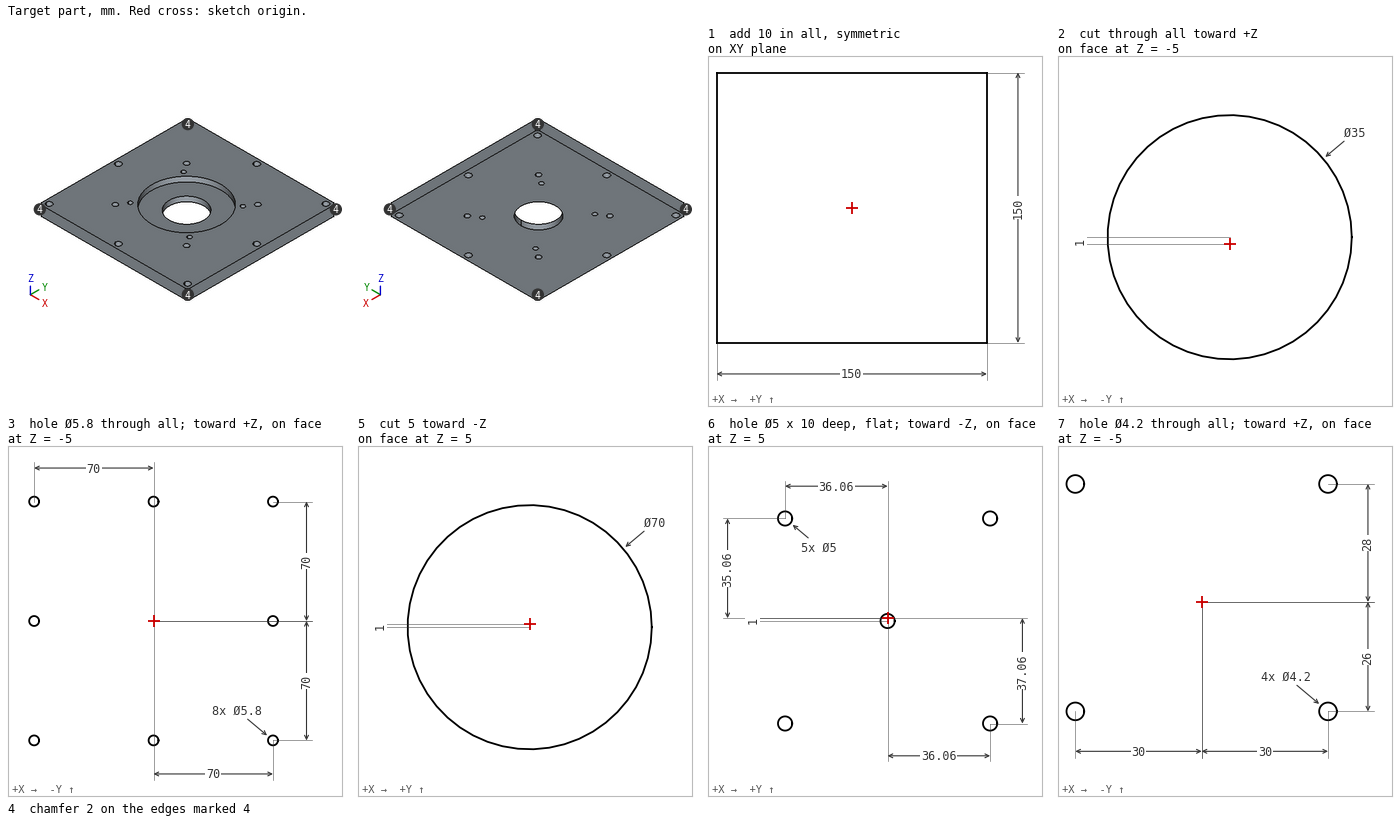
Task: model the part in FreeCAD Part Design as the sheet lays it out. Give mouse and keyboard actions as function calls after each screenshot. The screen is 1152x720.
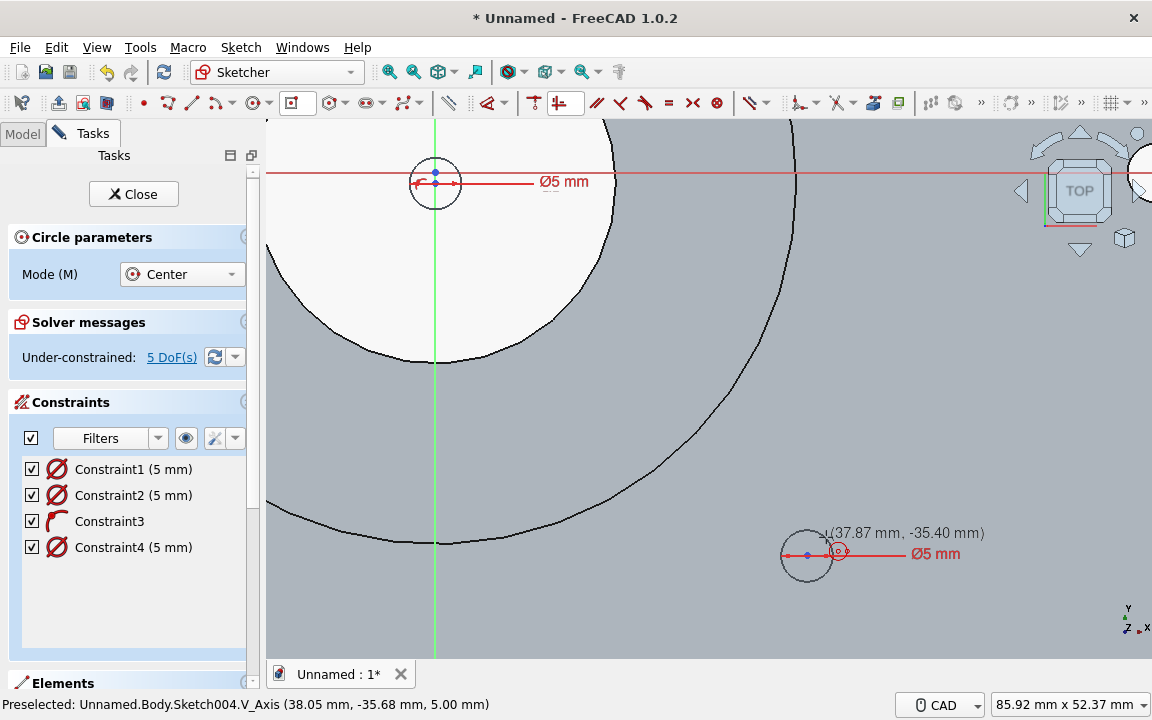
scroll(808, 557, down, 4)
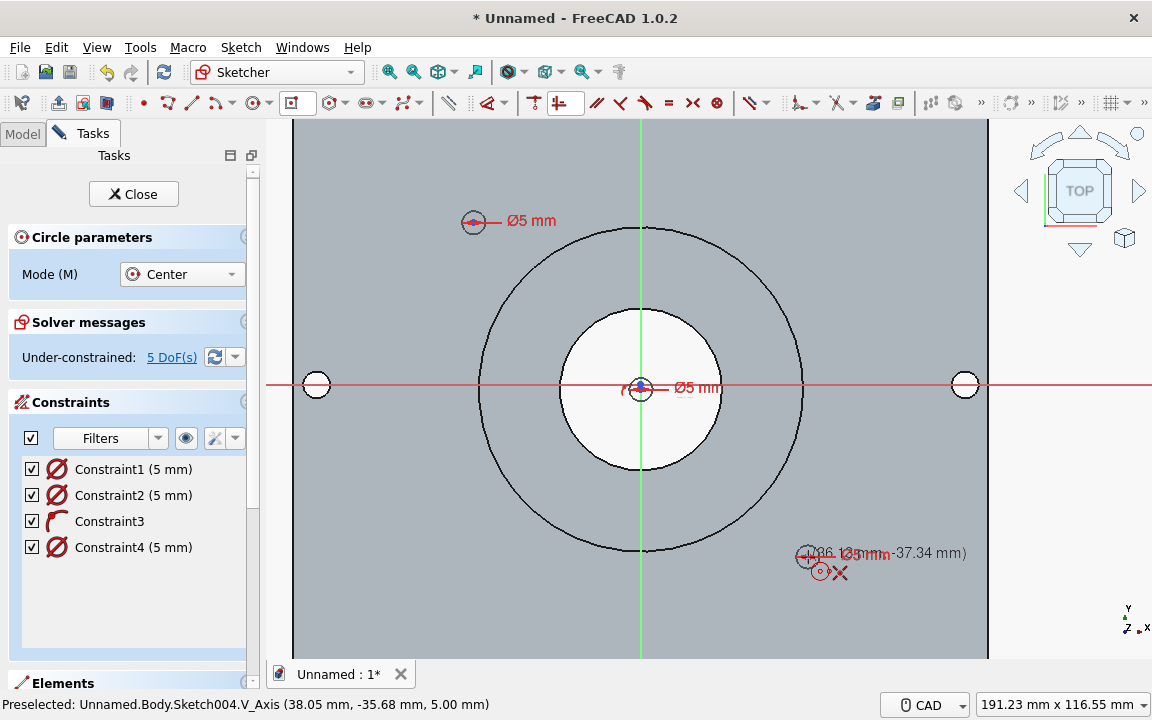
scroll(808, 222, up, 4)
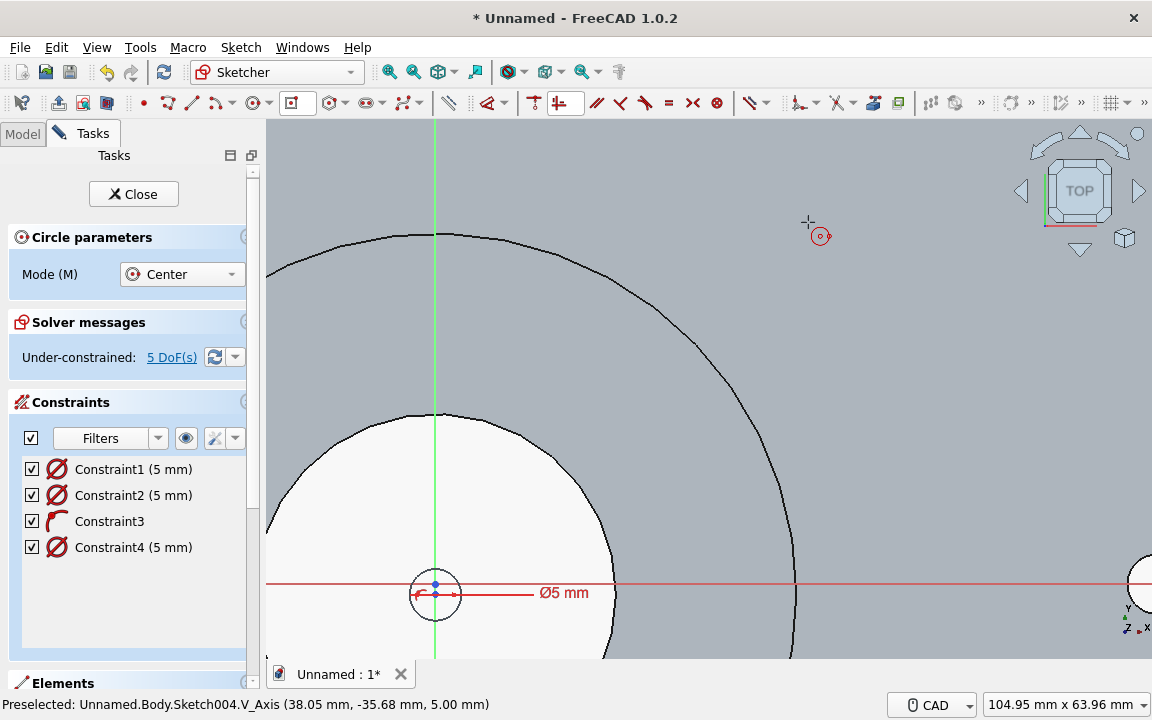
click(807, 223)
move(826, 205)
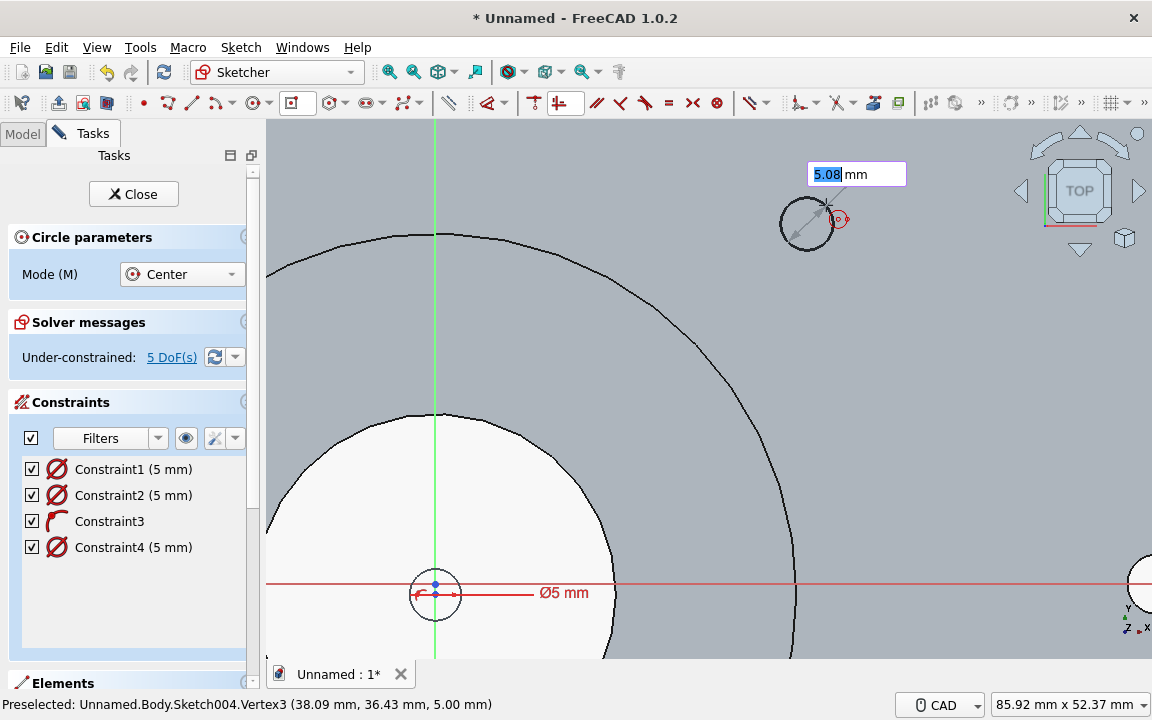
text(5)
key(Return)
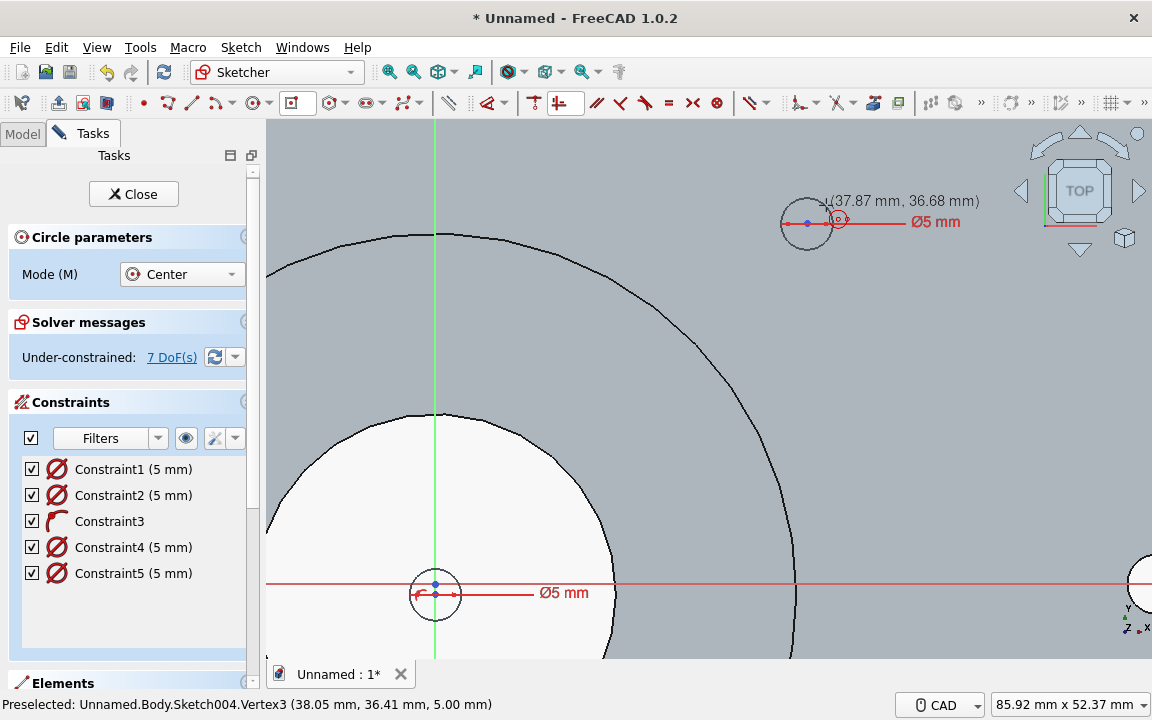
scroll(808, 221, down, 4)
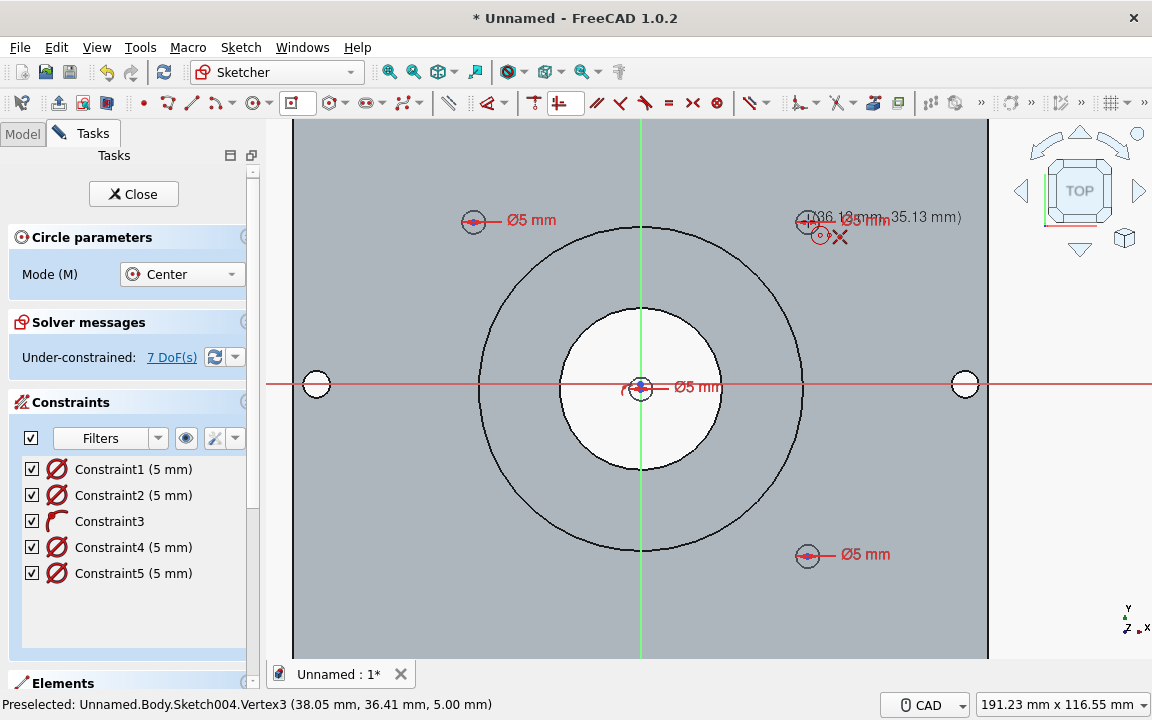
scroll(474, 556, up, 4)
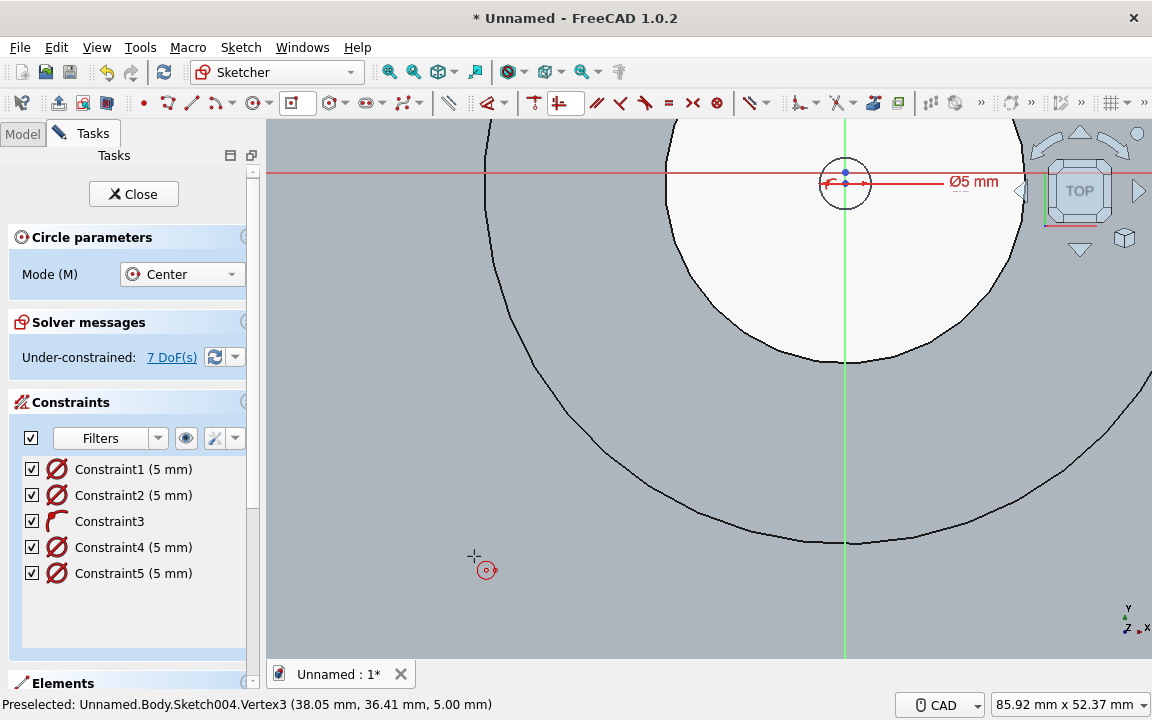
click(473, 555)
move(492, 537)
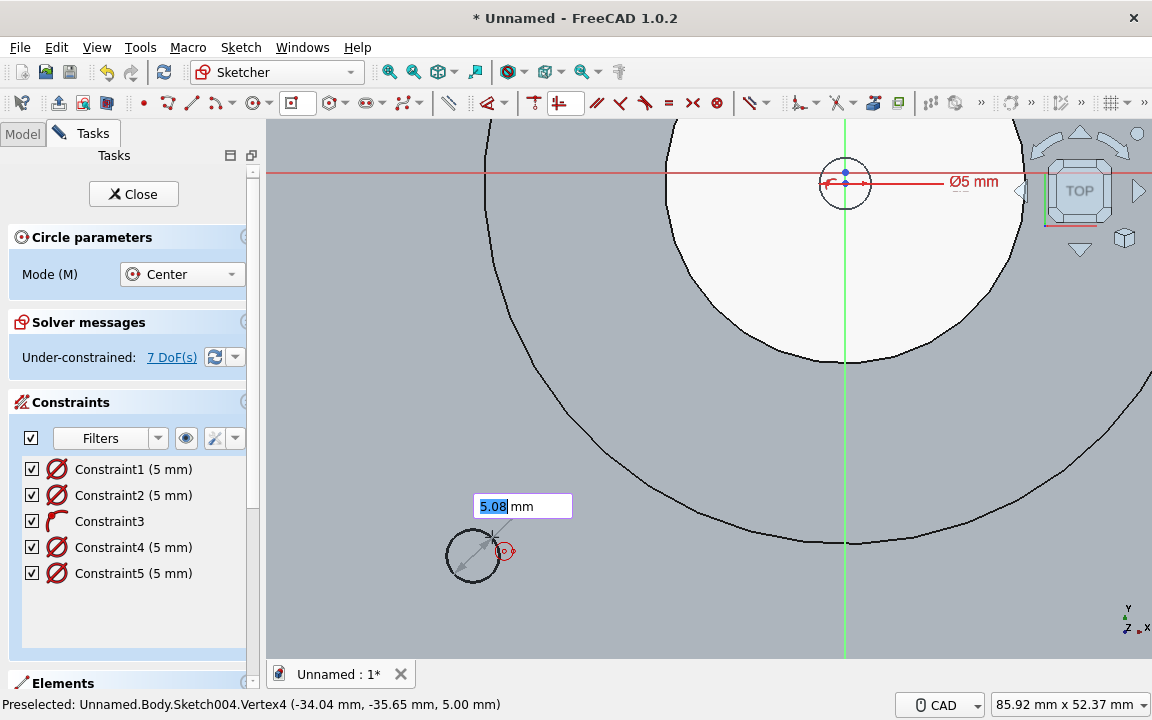
text(5)
key(Return)
key(Escape)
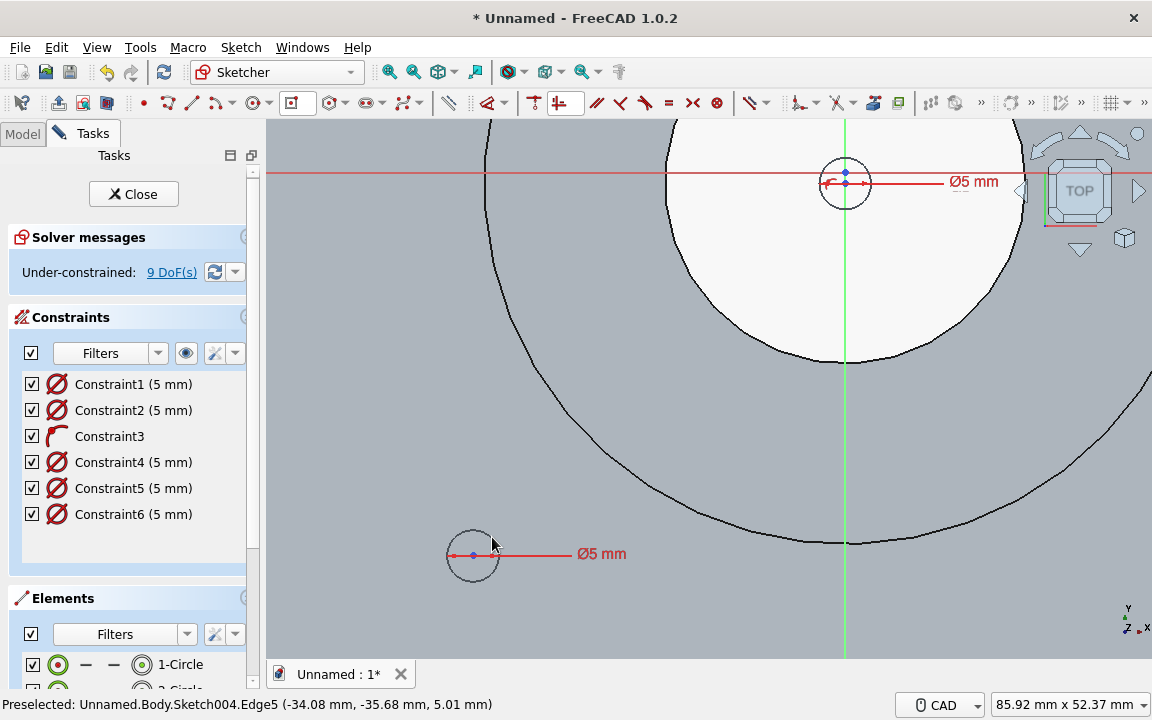
scroll(473, 557, down, 4)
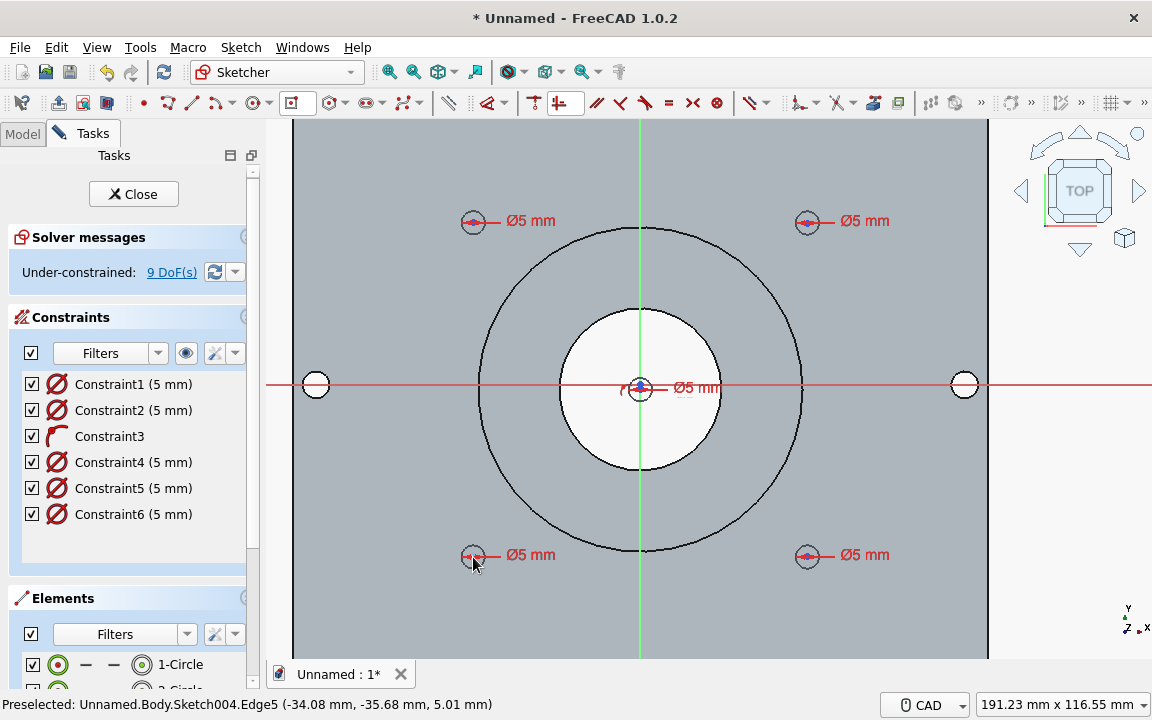
click(807, 557)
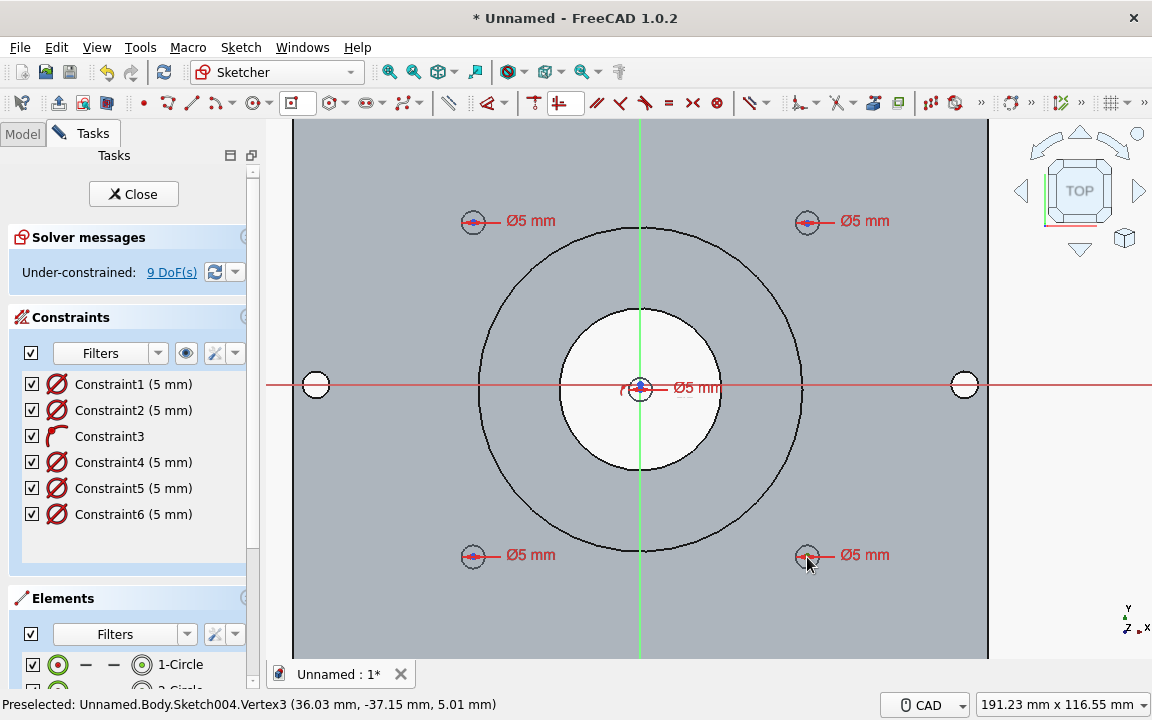
click(807, 223)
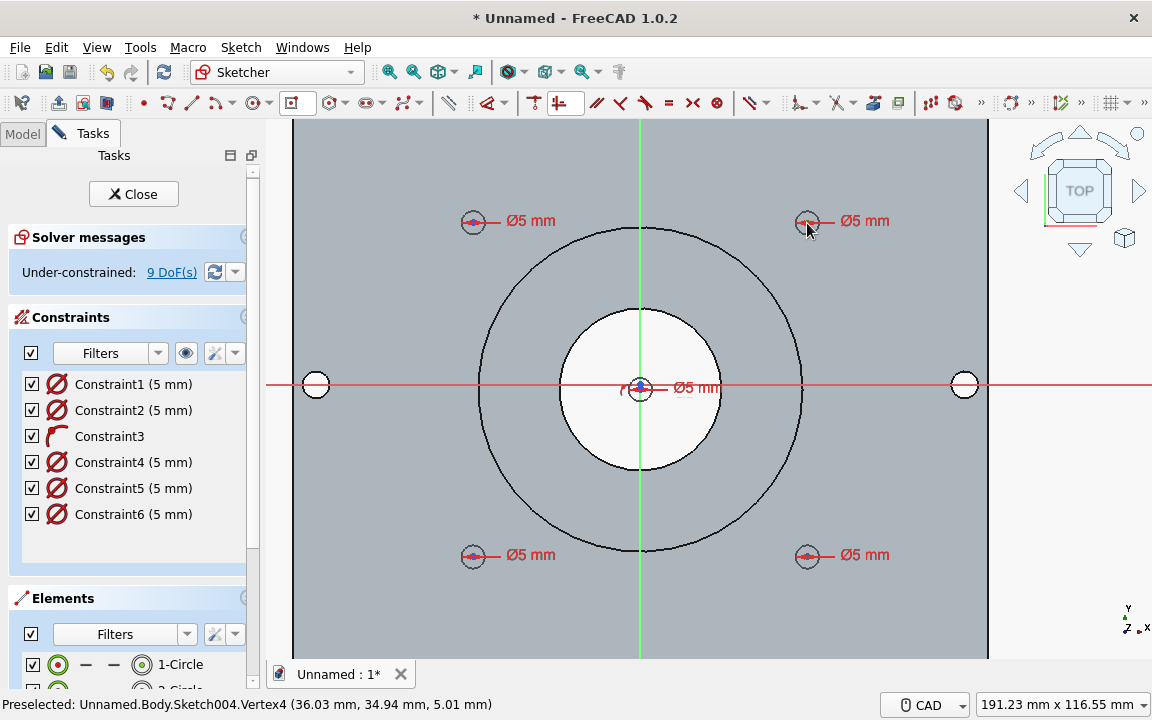
key(v)